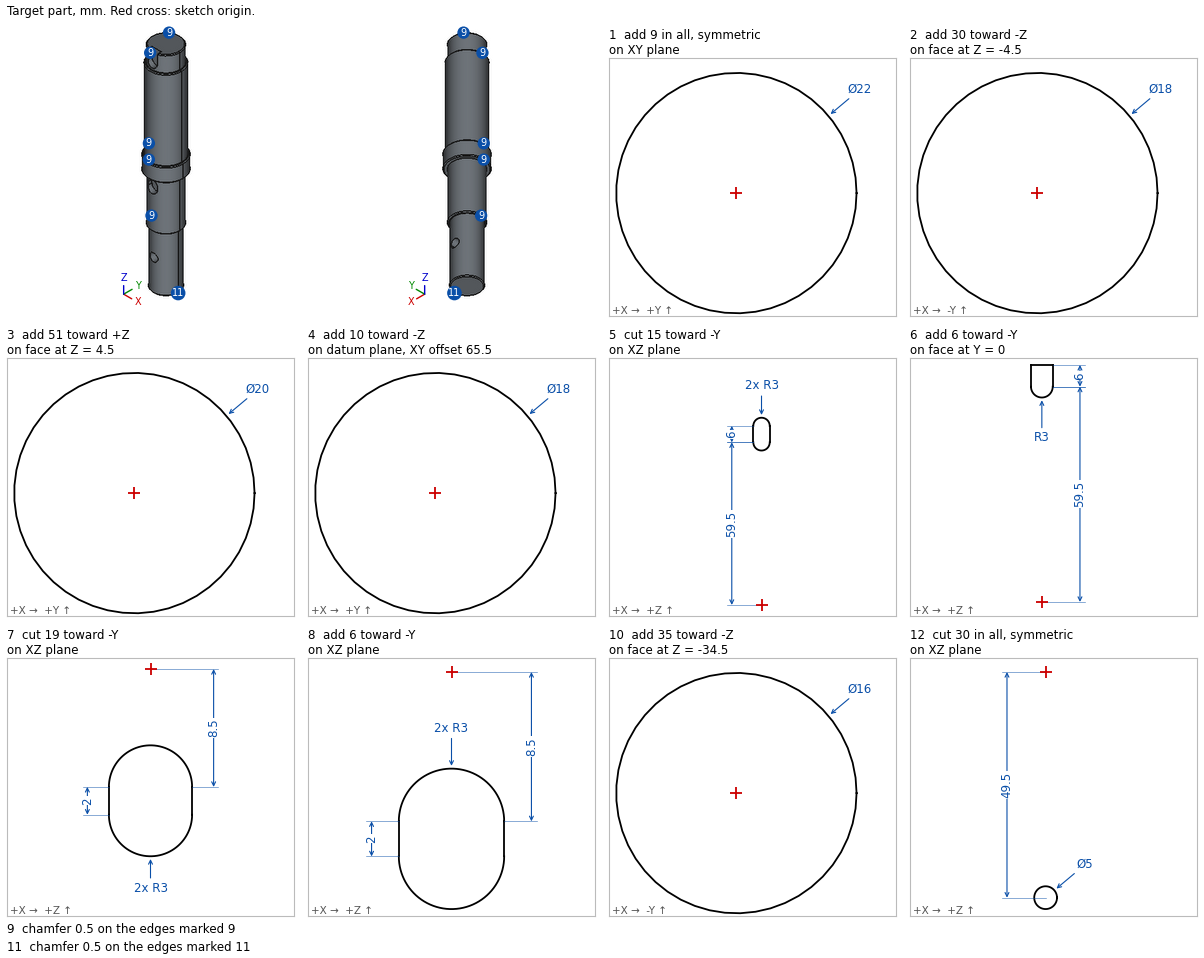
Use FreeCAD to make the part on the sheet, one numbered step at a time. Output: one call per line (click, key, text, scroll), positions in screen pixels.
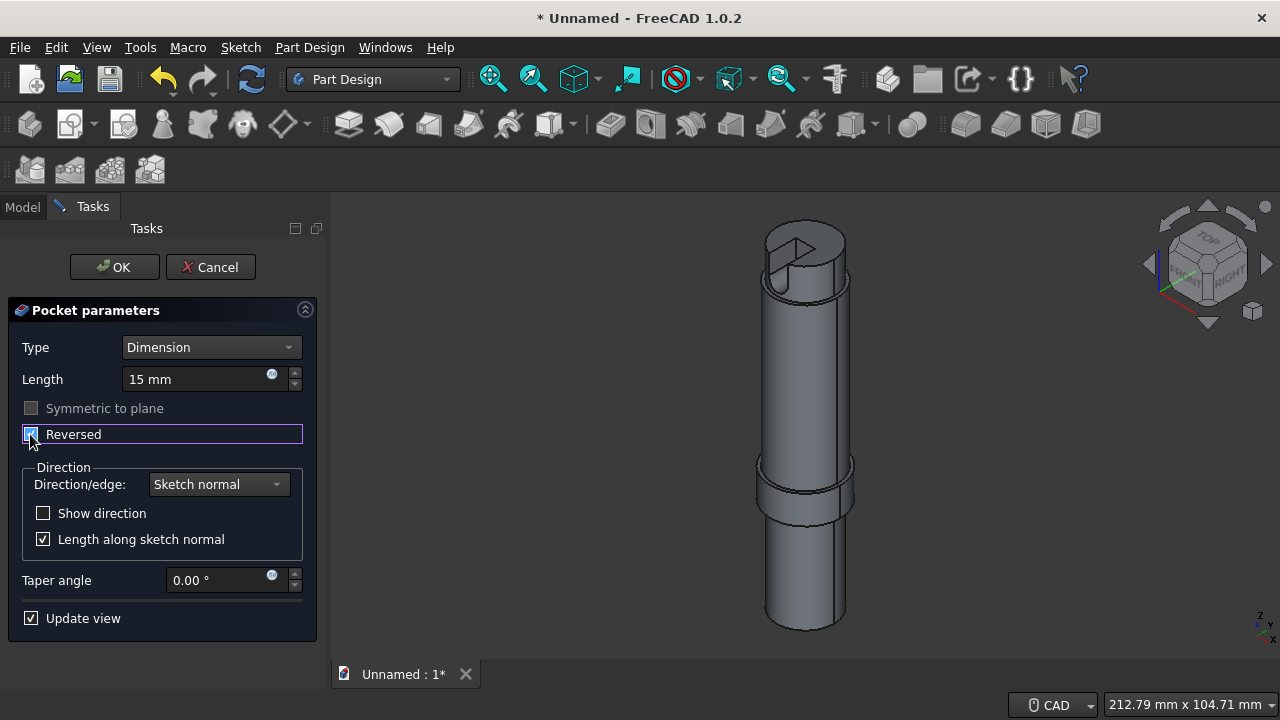
click(115, 267)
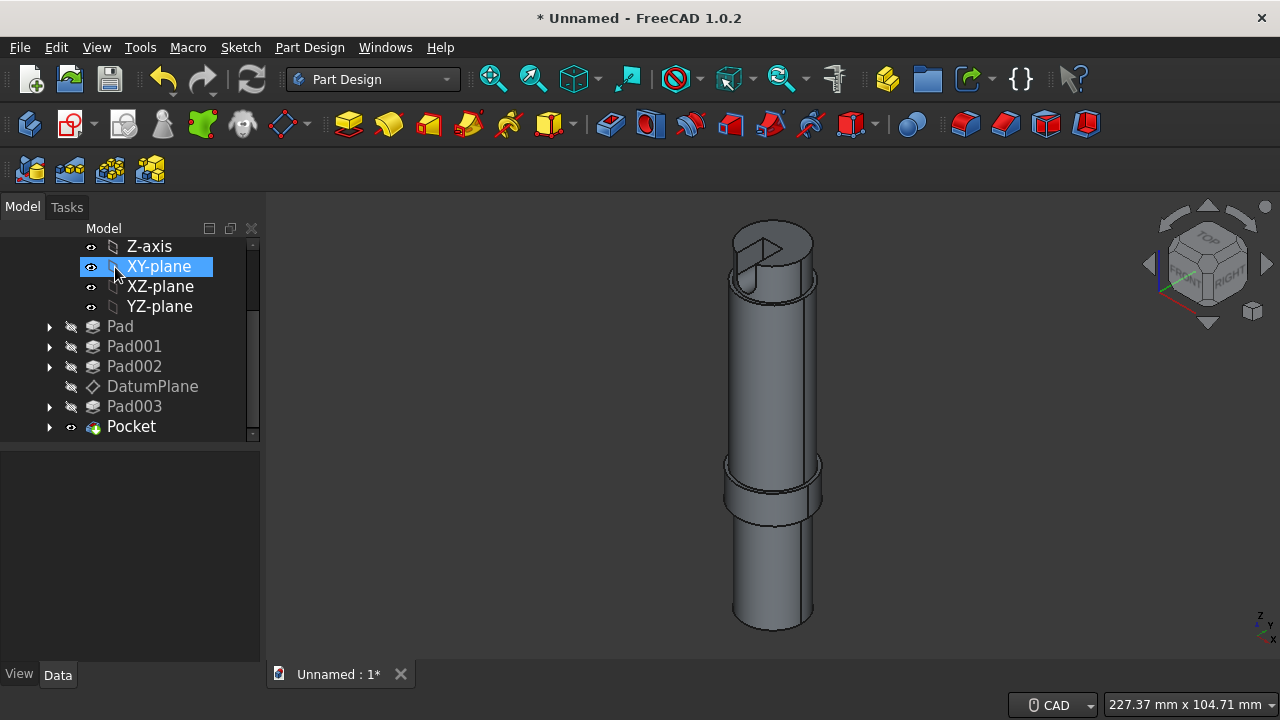
key(1)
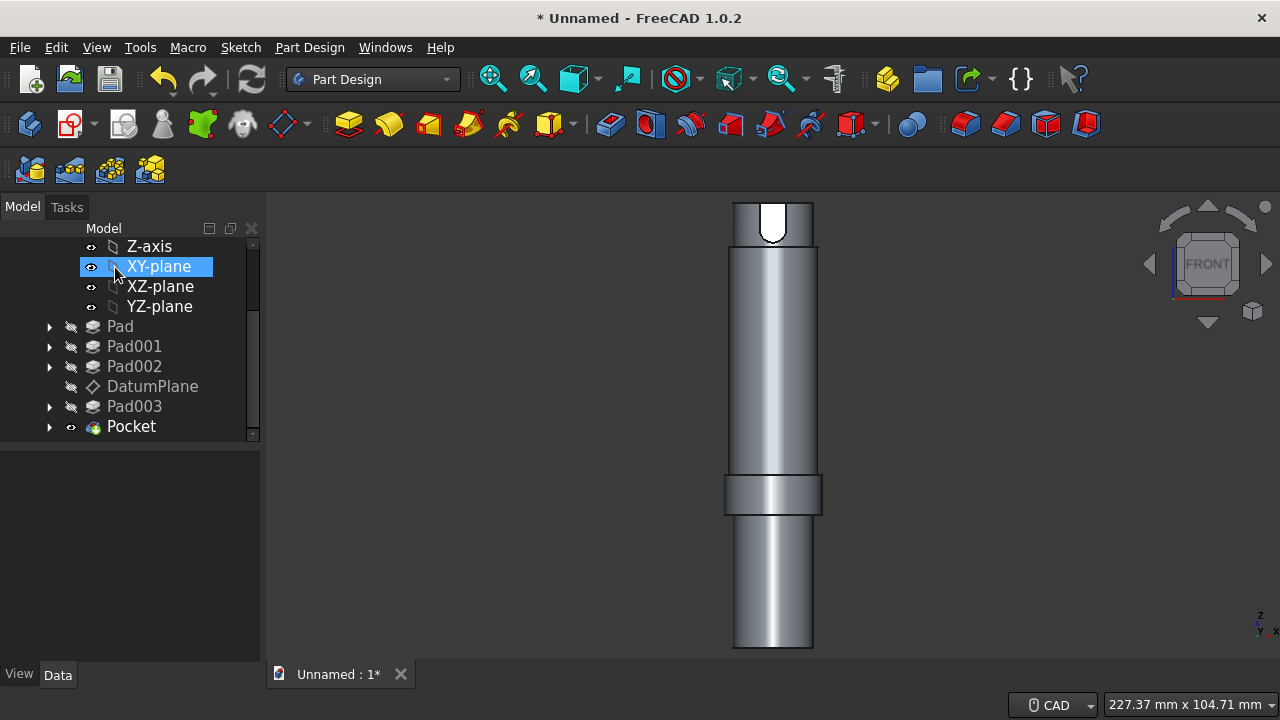
click(773, 222)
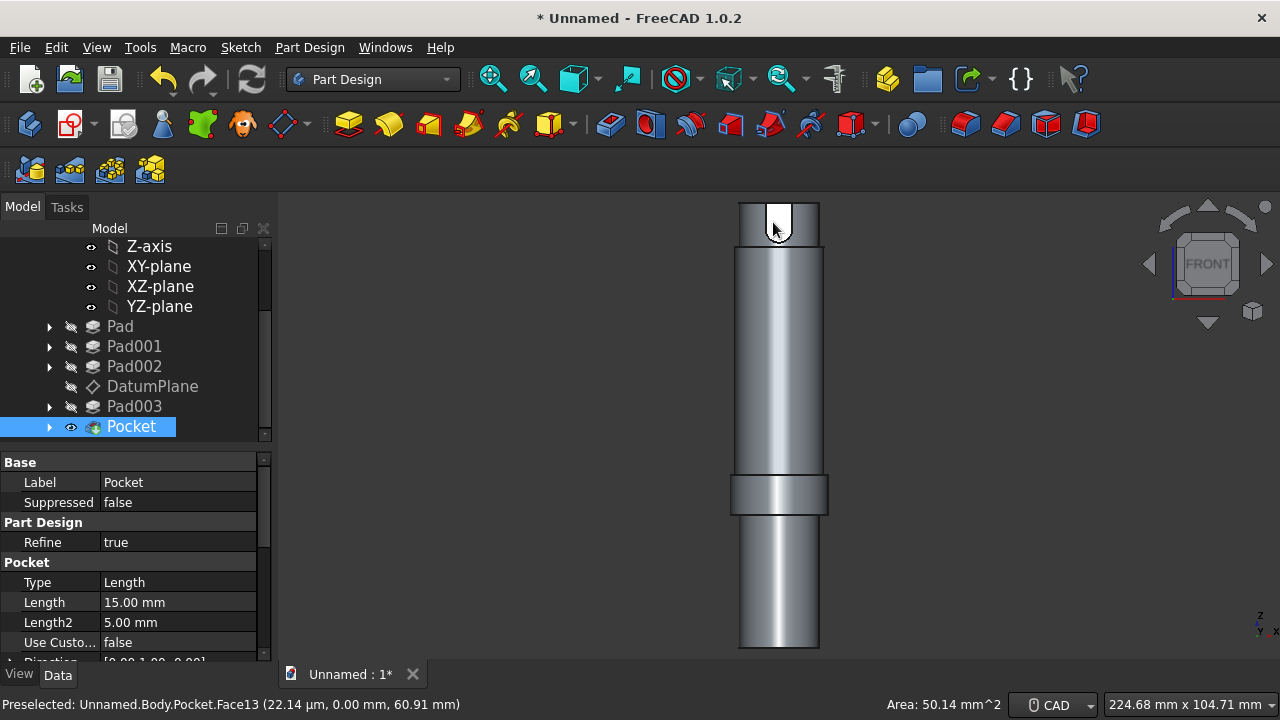
click(70, 124)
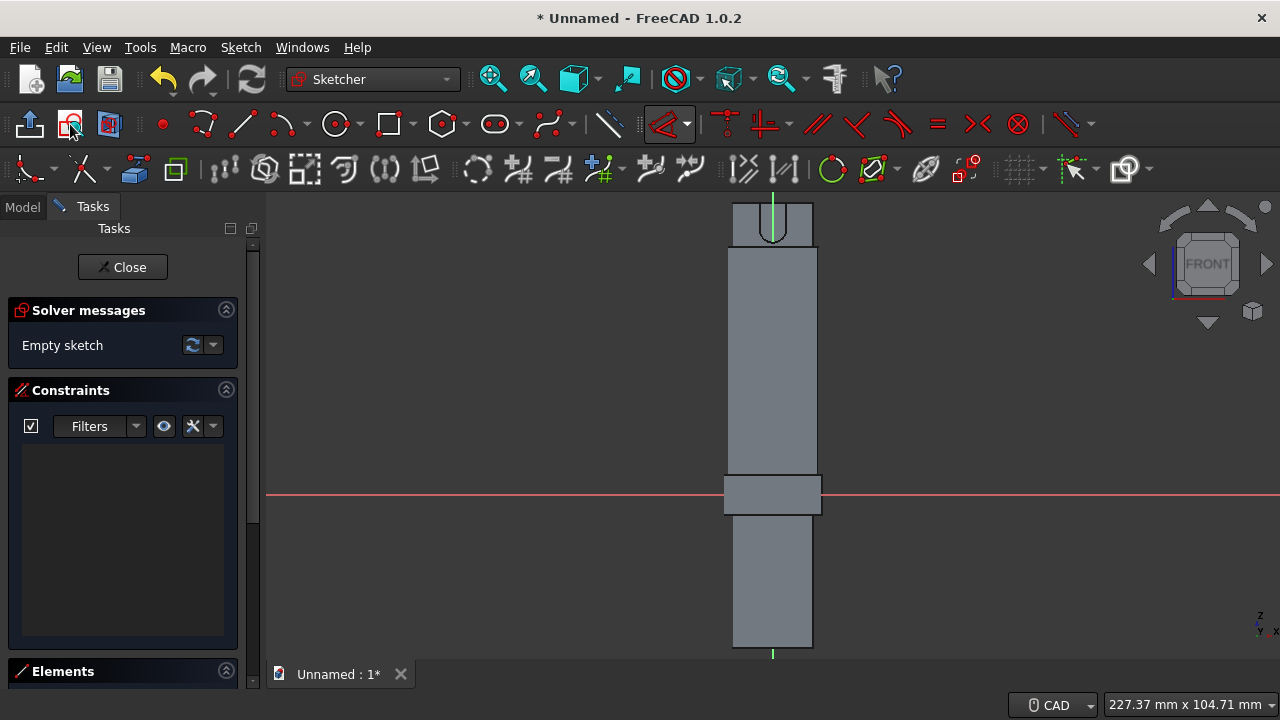
scroll(704, 426, down, 5)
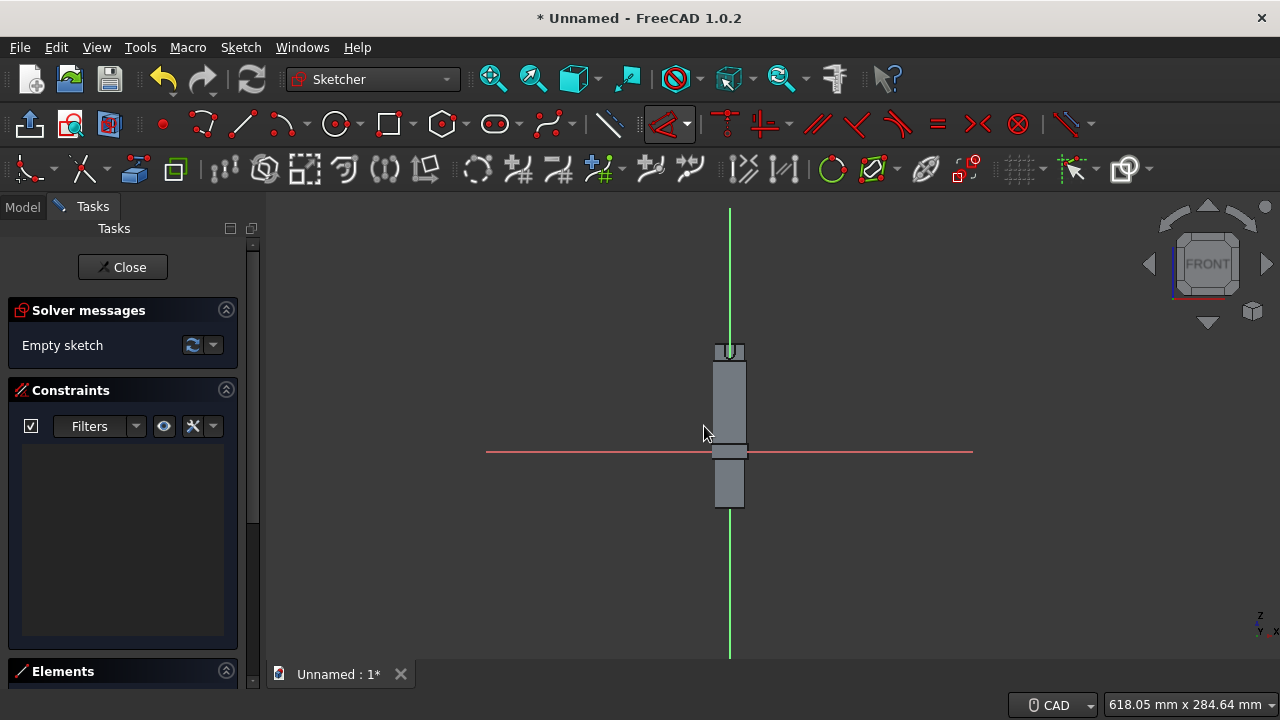
scroll(731, 348, up, 15)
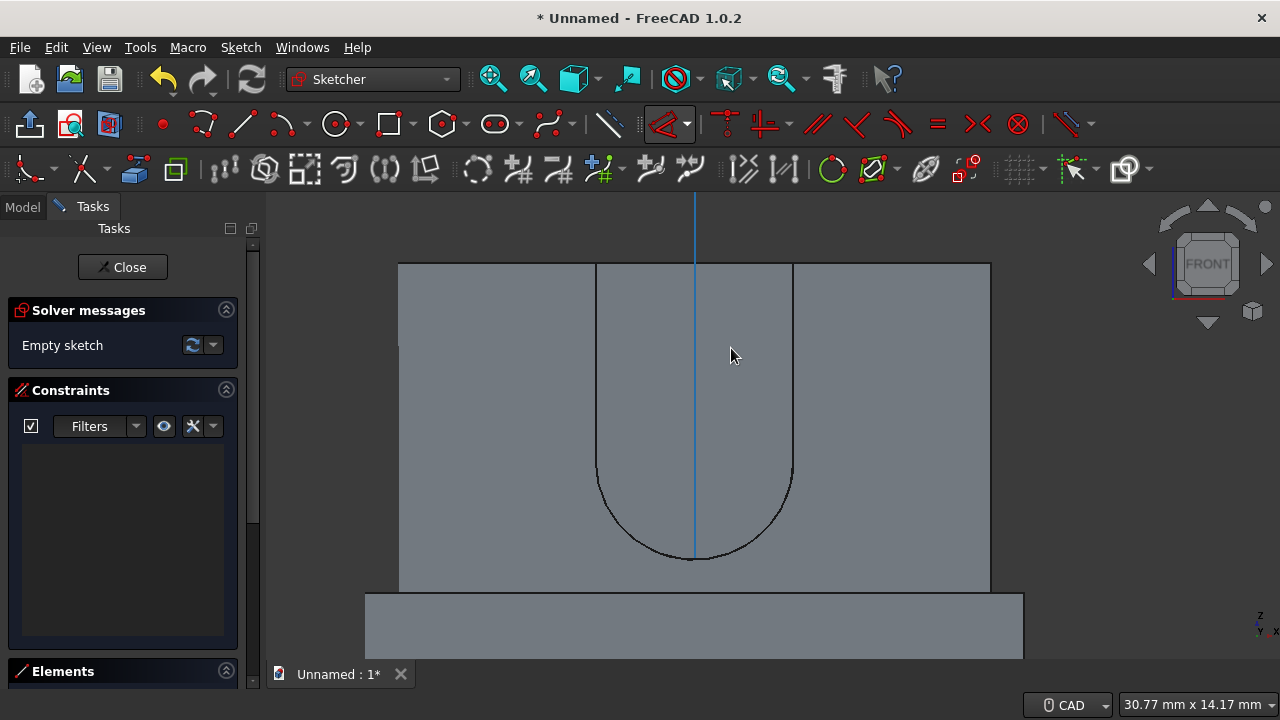
click(204, 124)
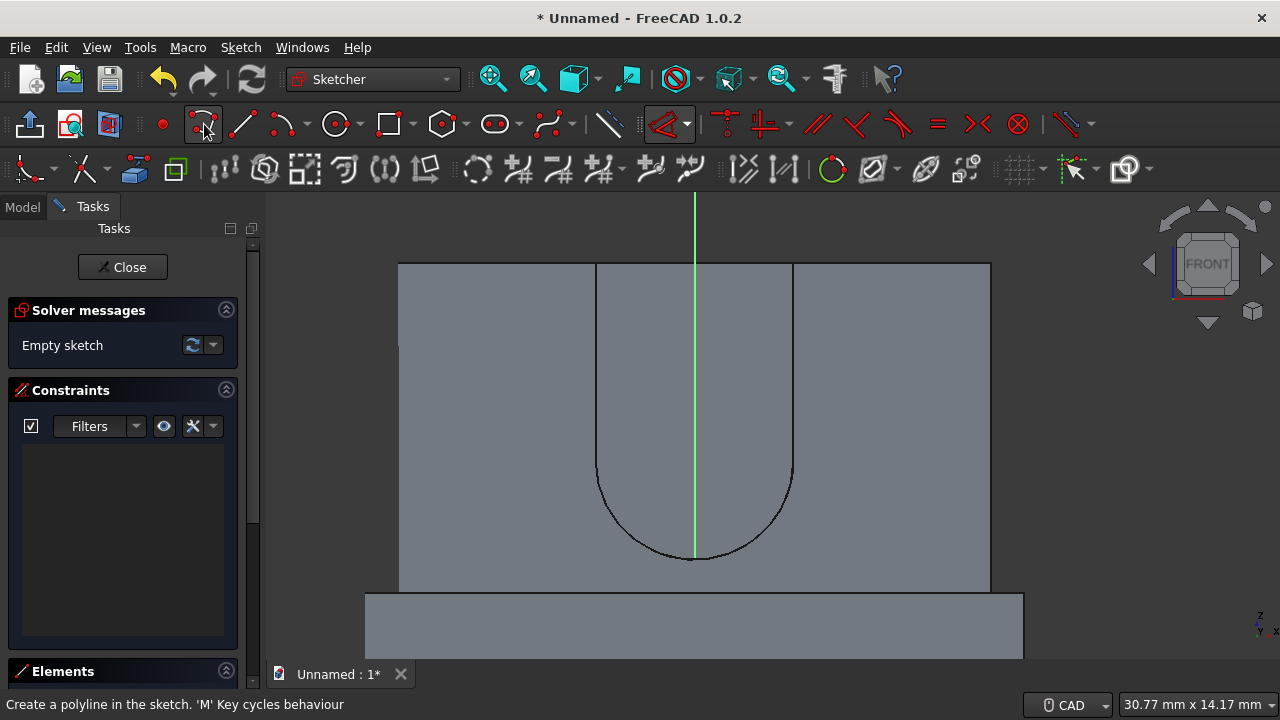
click(793, 461)
click(793, 263)
click(596, 263)
click(596, 461)
right_click(596, 461)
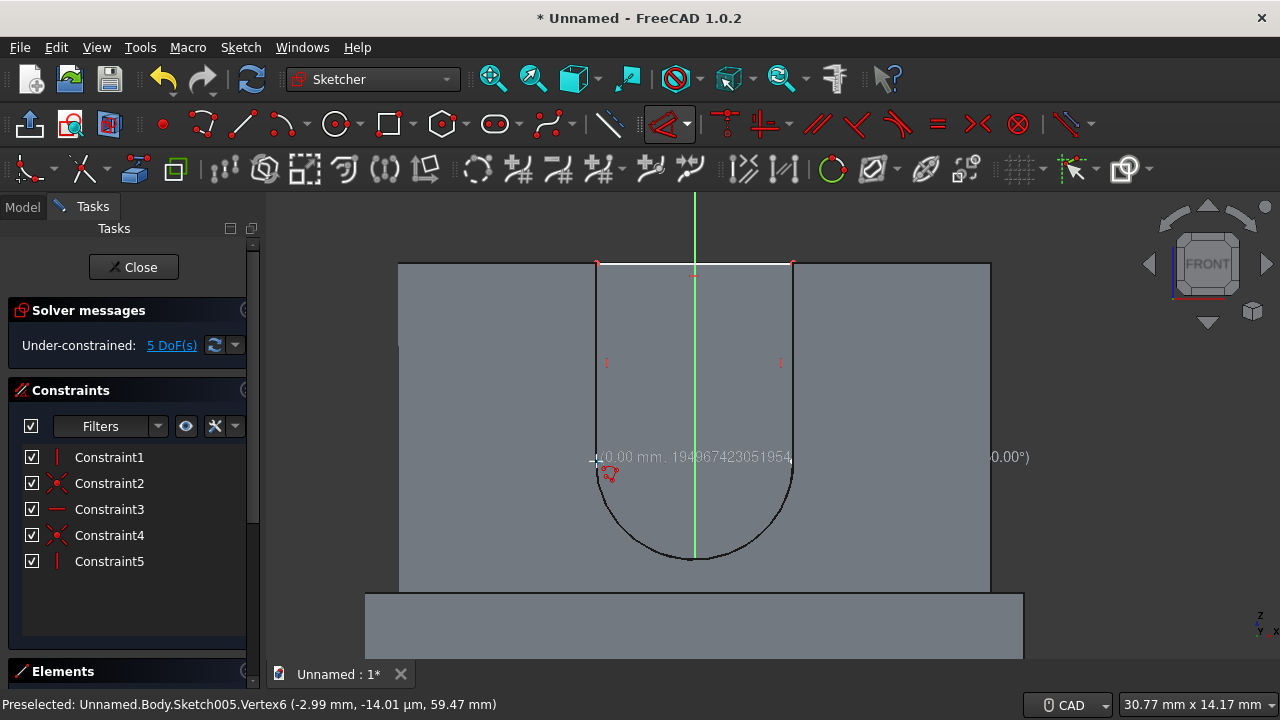
key(g)
key(3)
key(a)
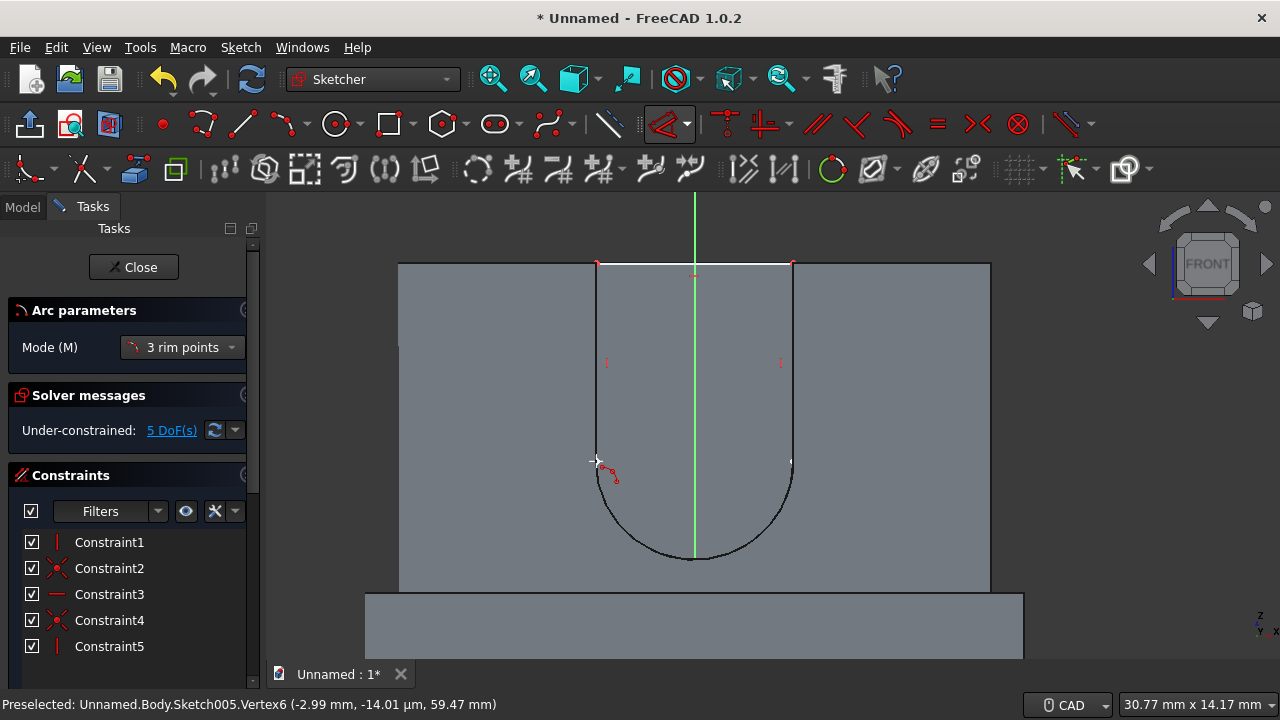
click(596, 462)
click(793, 462)
click(664, 555)
key(Escape)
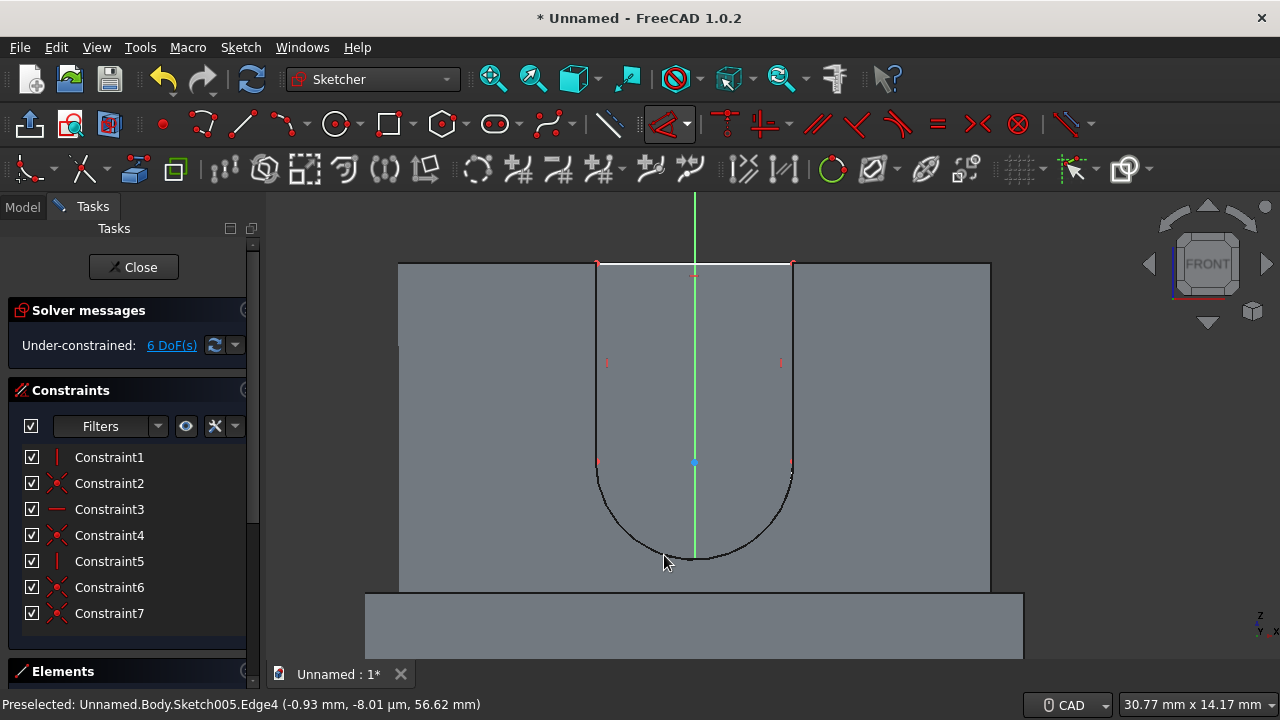
click(793, 403)